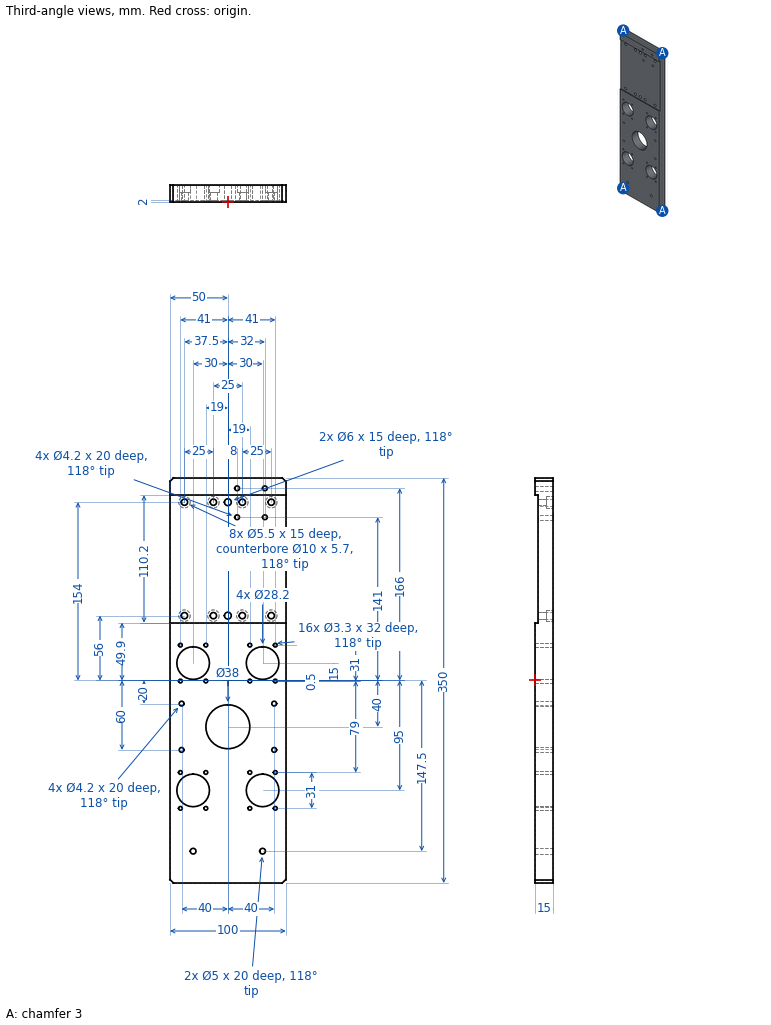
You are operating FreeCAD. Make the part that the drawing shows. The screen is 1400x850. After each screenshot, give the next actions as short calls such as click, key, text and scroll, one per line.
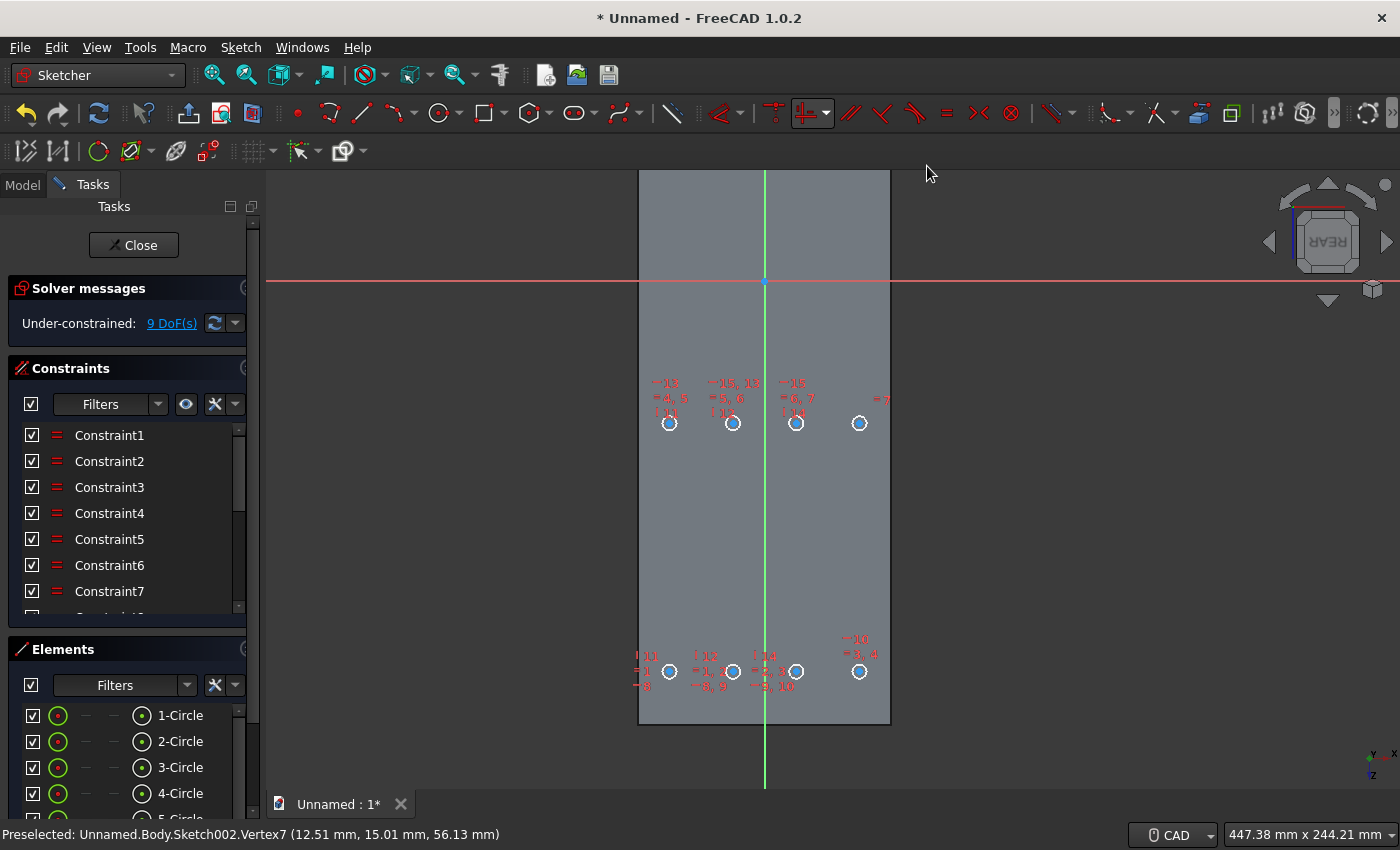
click(860, 672)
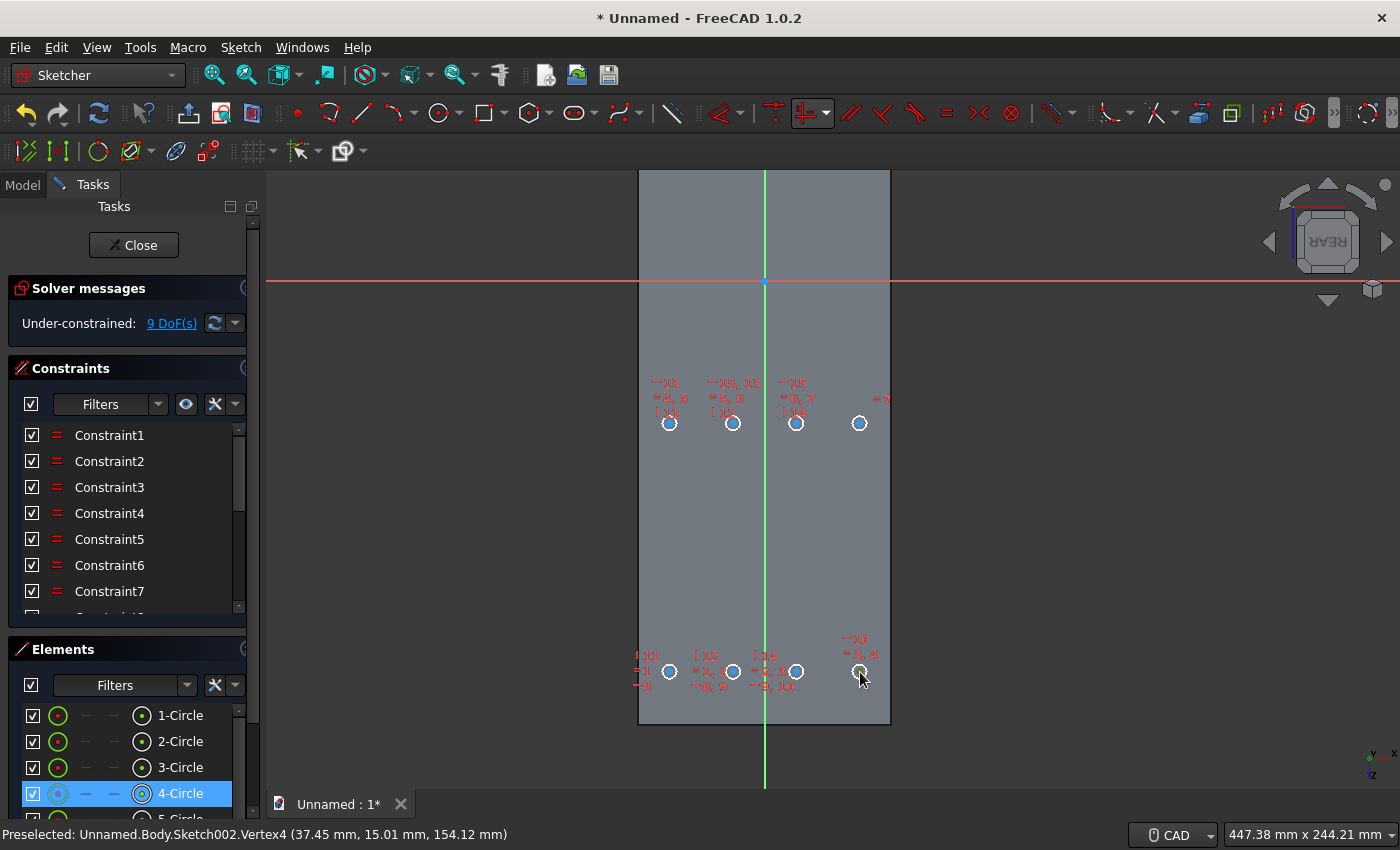
click(860, 423)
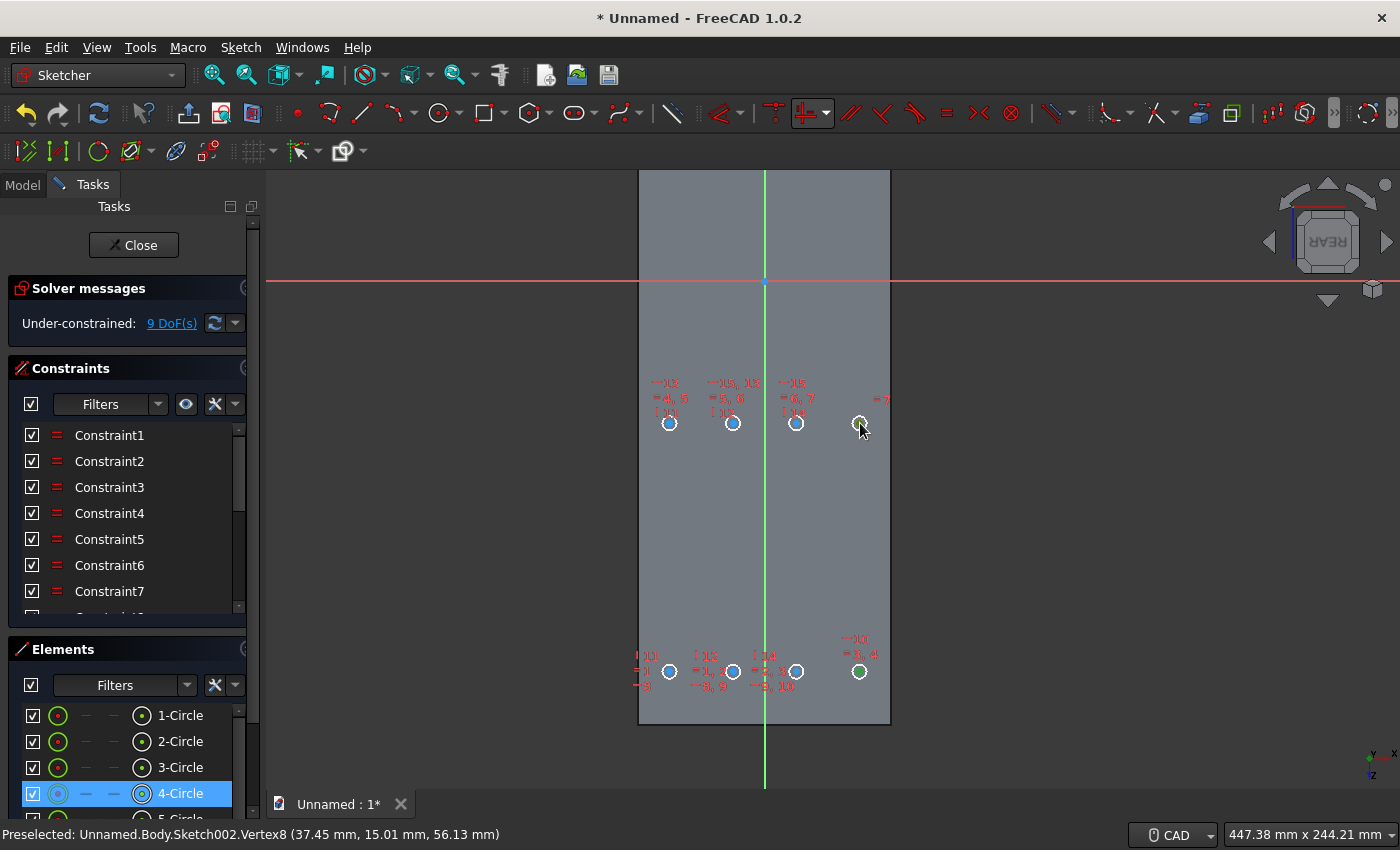
key(v)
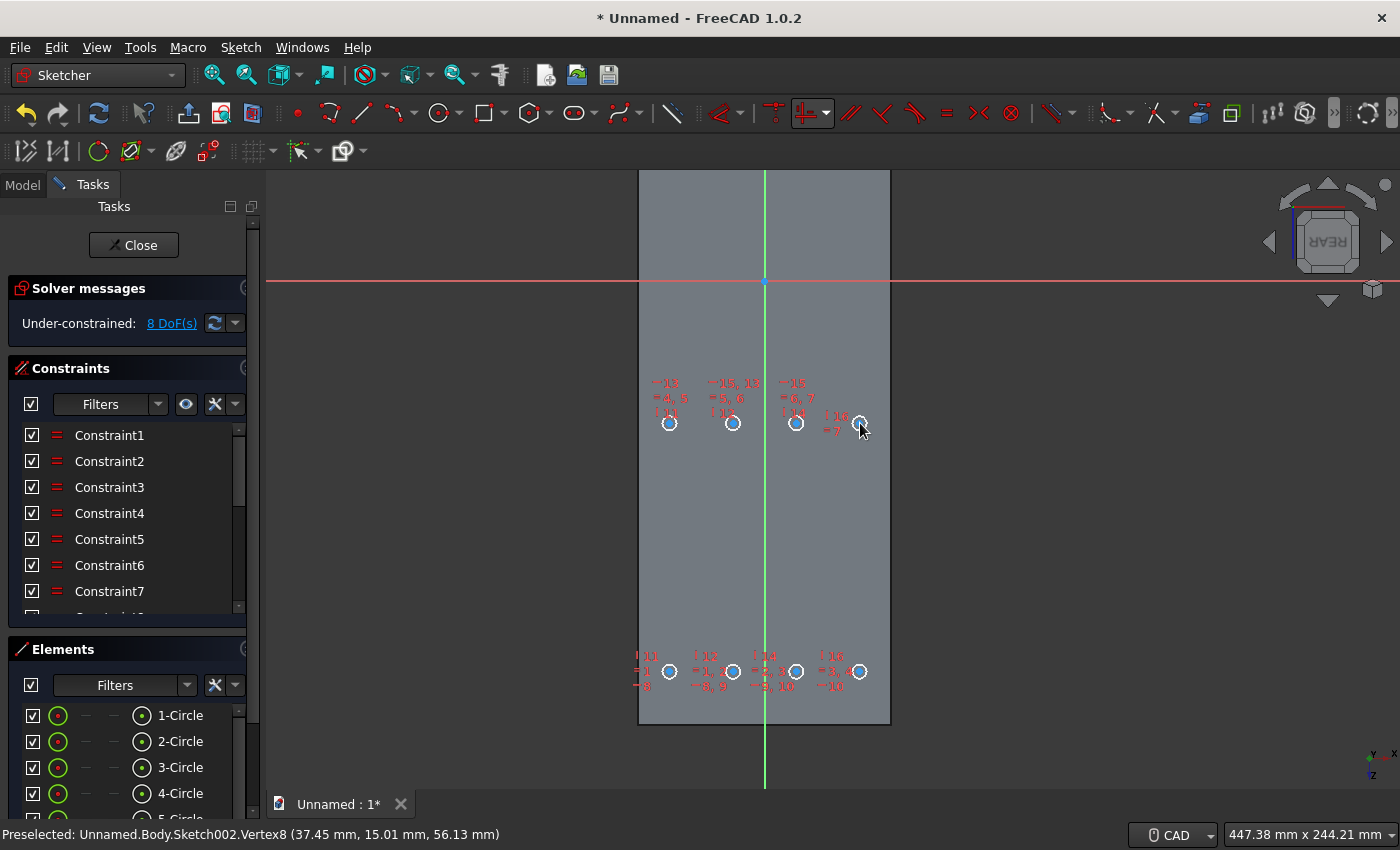
click(796, 423)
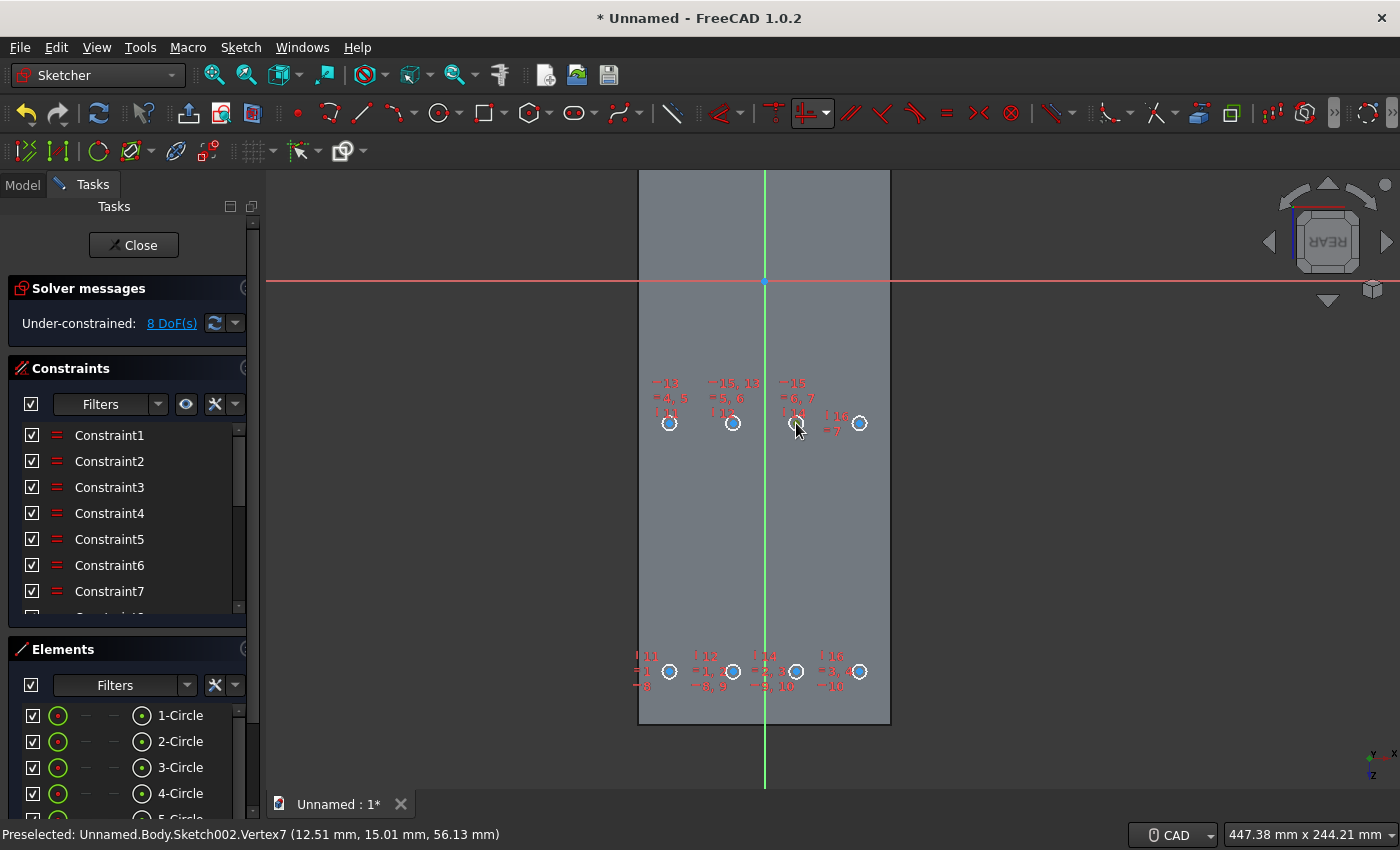
click(860, 423)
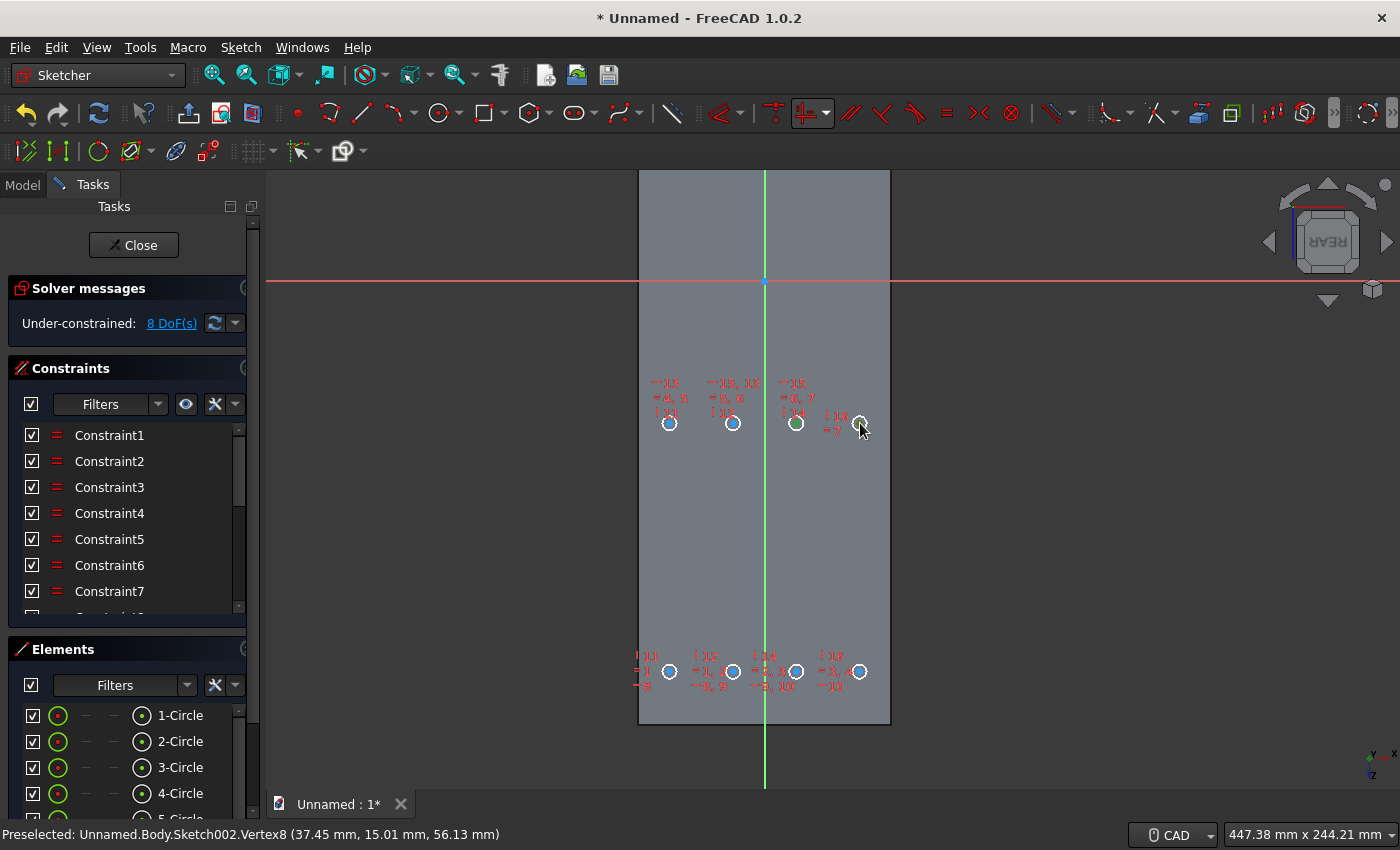
key(h)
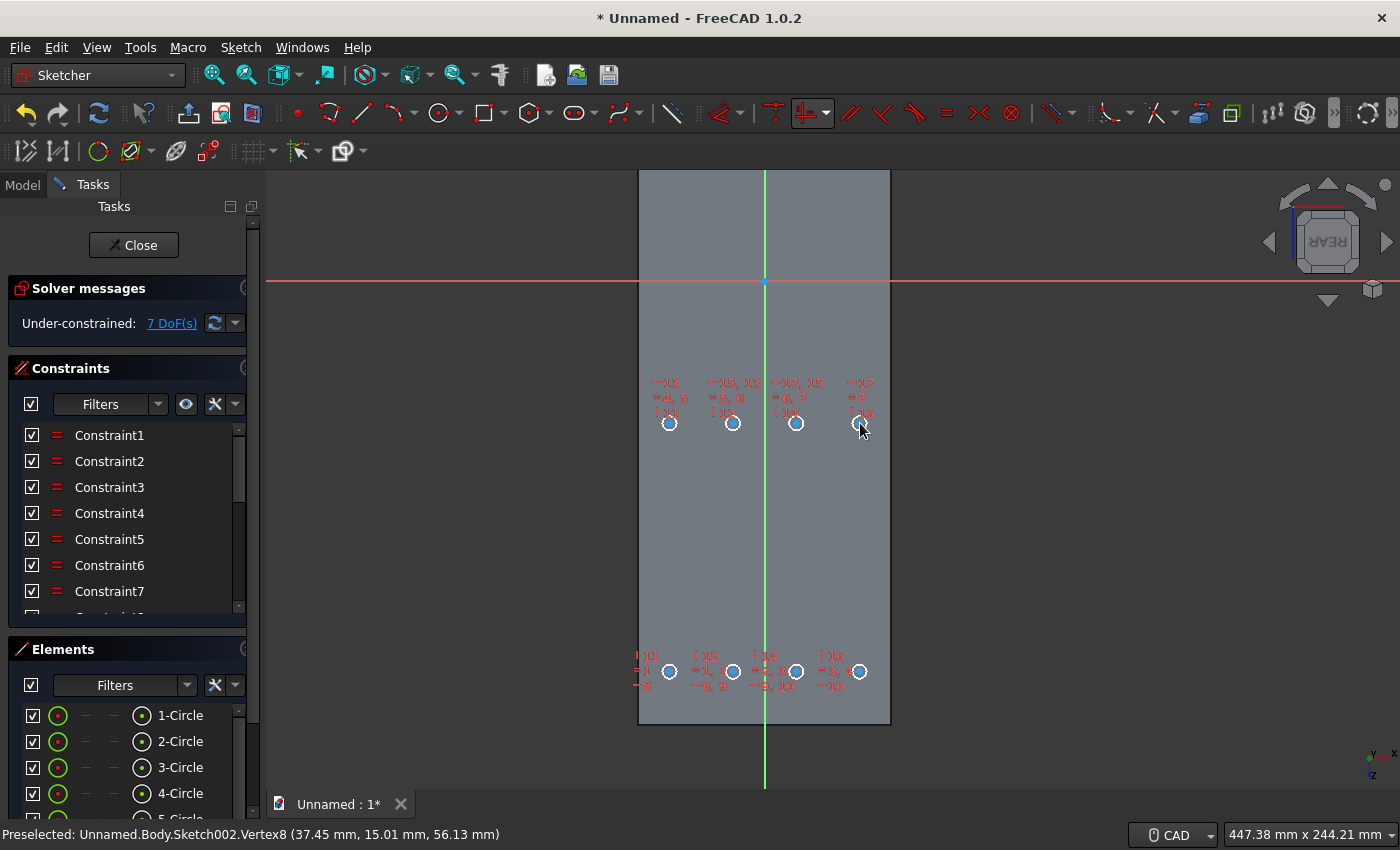
click(720, 114)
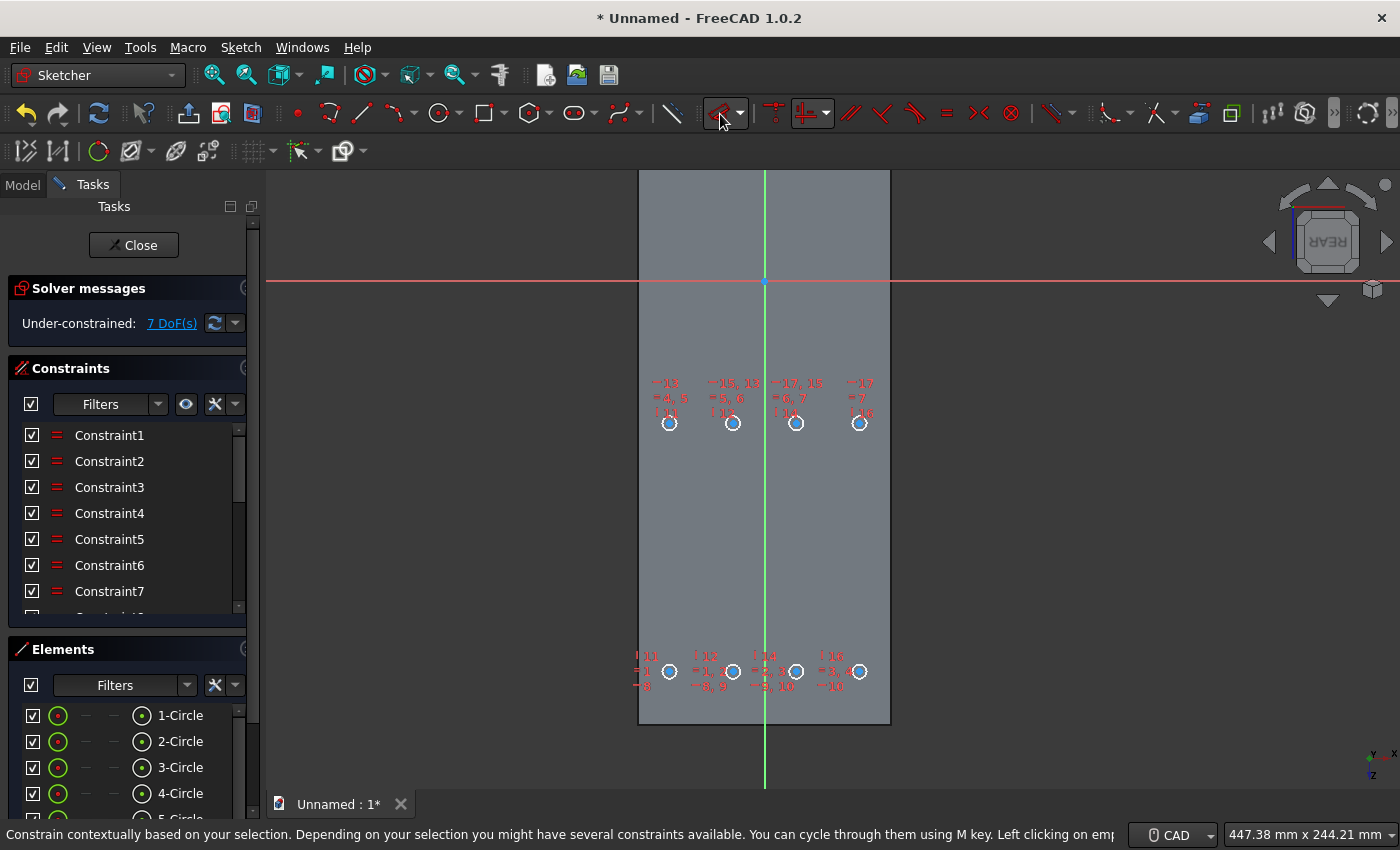
scroll(665, 667, up, 6)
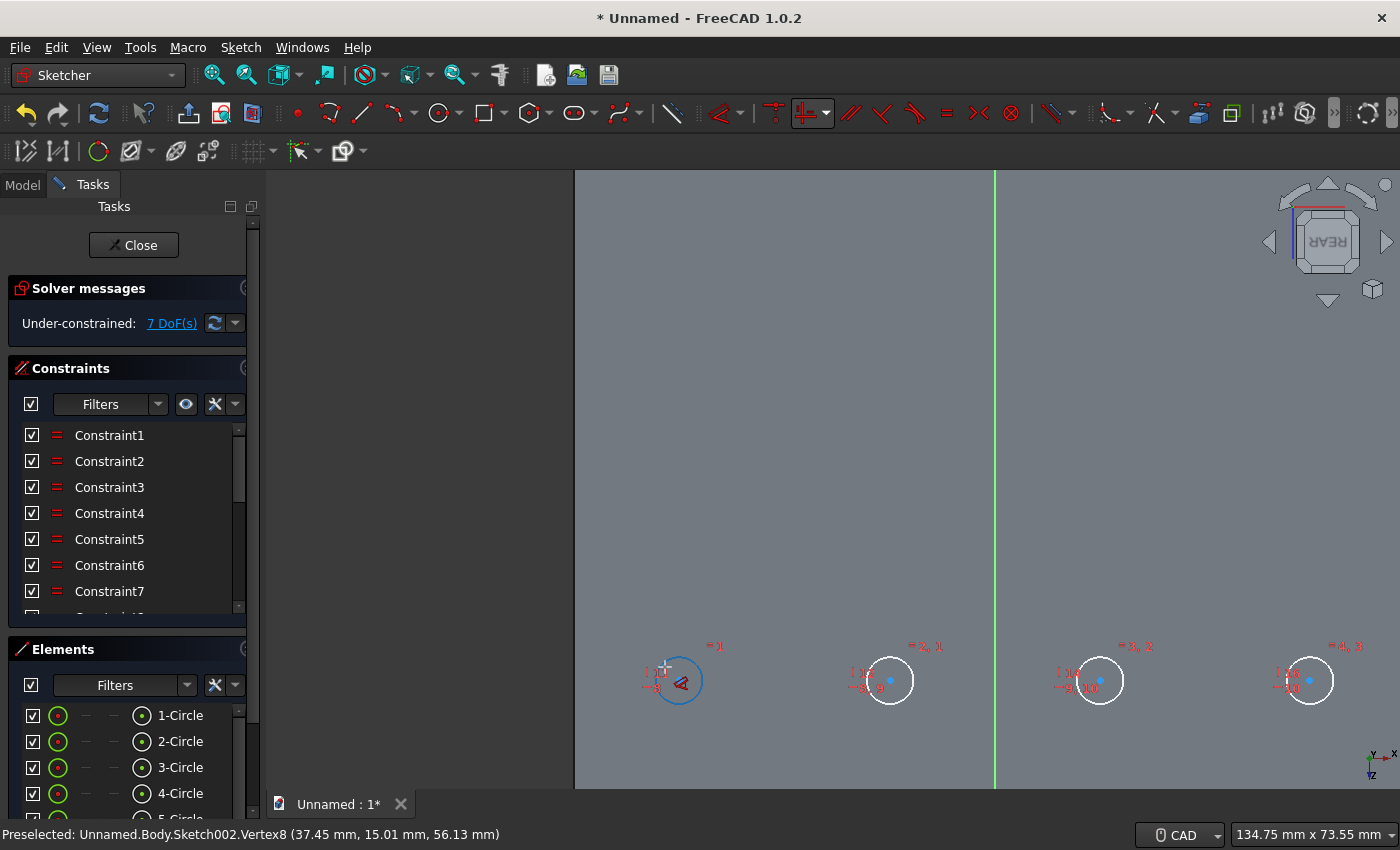
click(663, 664)
click(641, 641)